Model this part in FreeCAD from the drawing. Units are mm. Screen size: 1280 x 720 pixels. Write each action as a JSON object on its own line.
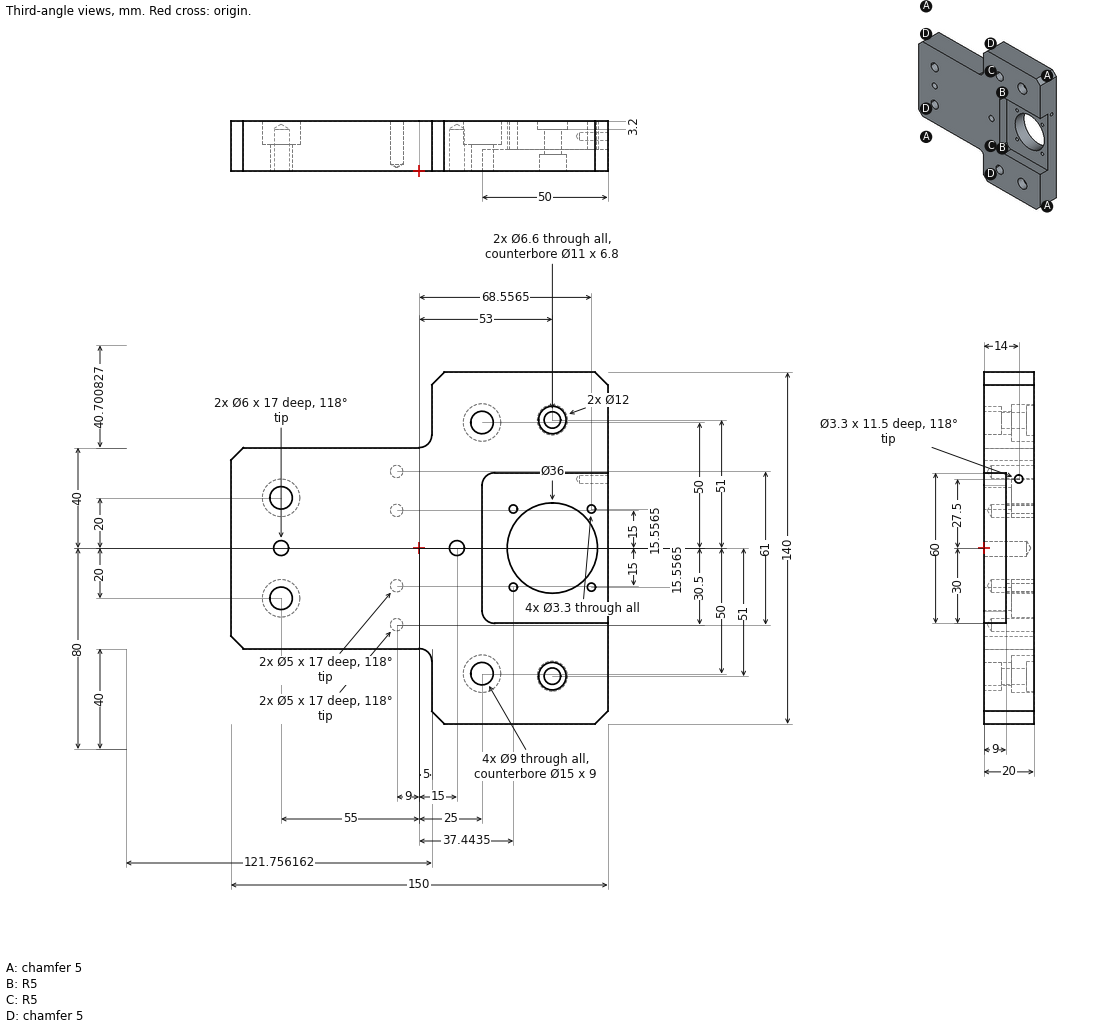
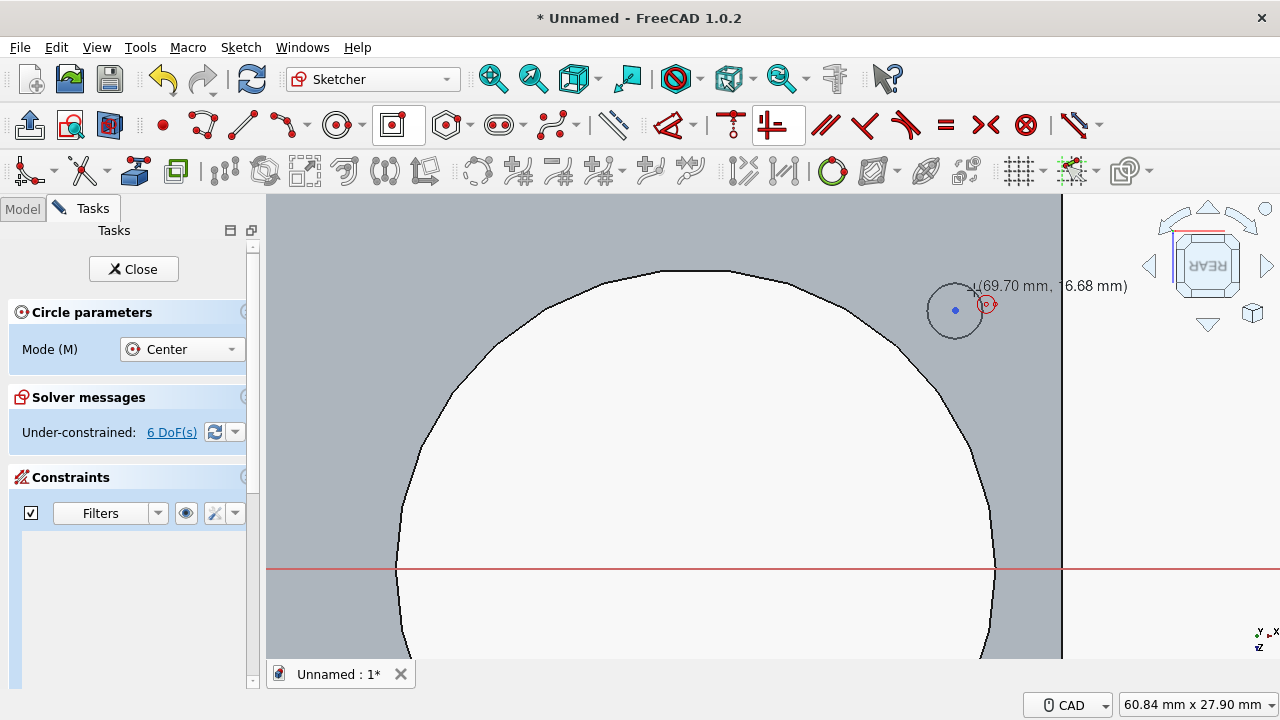
{"action": "left_click", "coordinate": [436, 310]}
{"action": "left_click", "coordinate": [456, 290]}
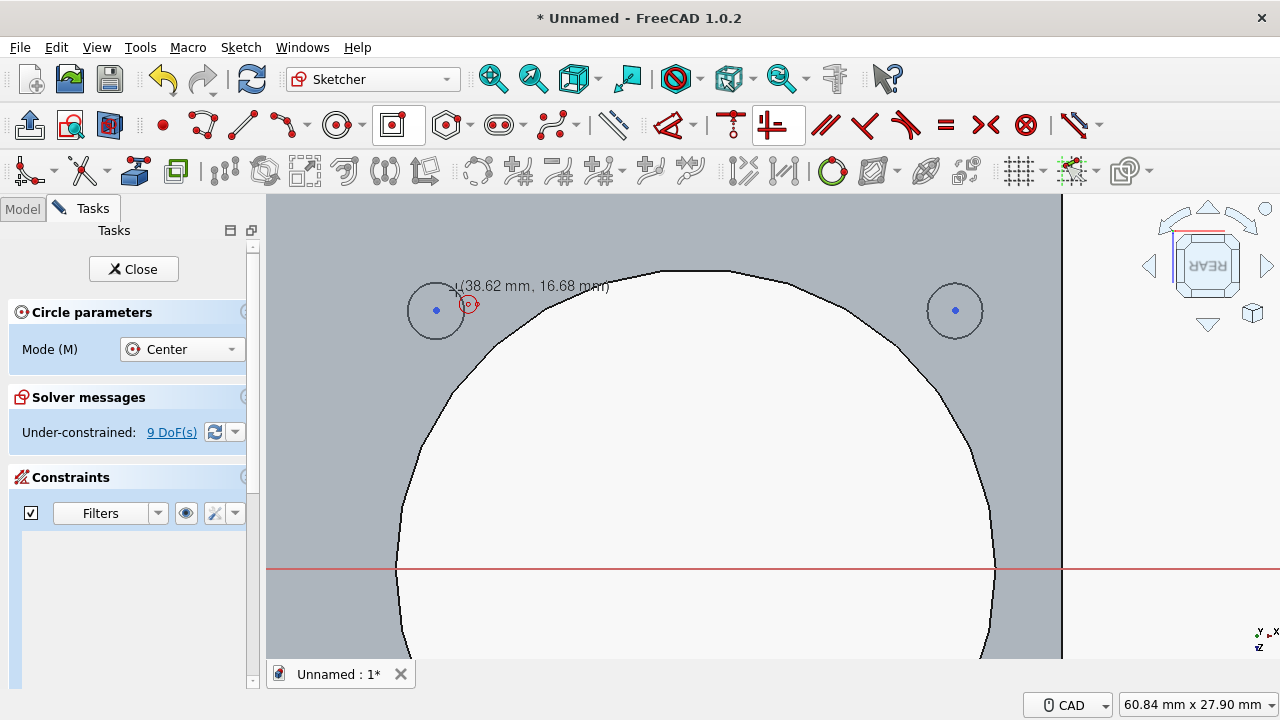
{"action": "scroll", "coordinate": [955, 310], "scroll_direction": "down", "scroll_amount": 4}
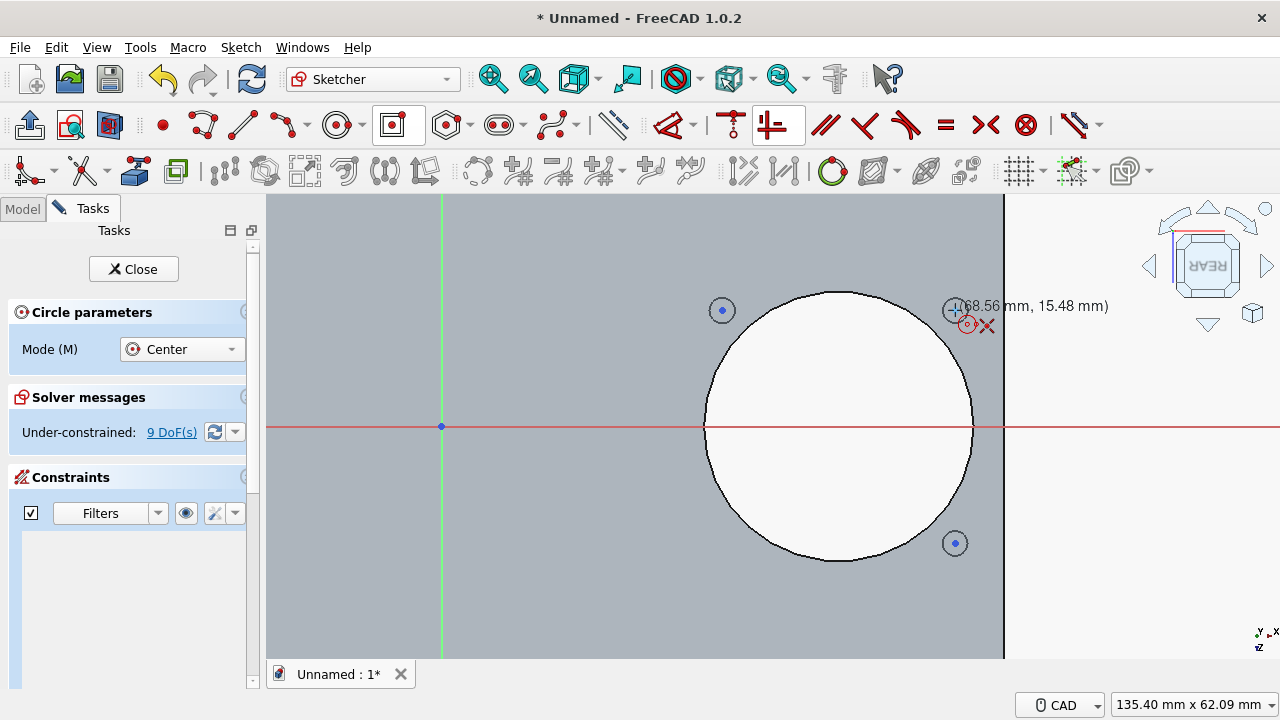
{"action": "scroll", "coordinate": [722, 543], "scroll_direction": "up", "scroll_amount": 4}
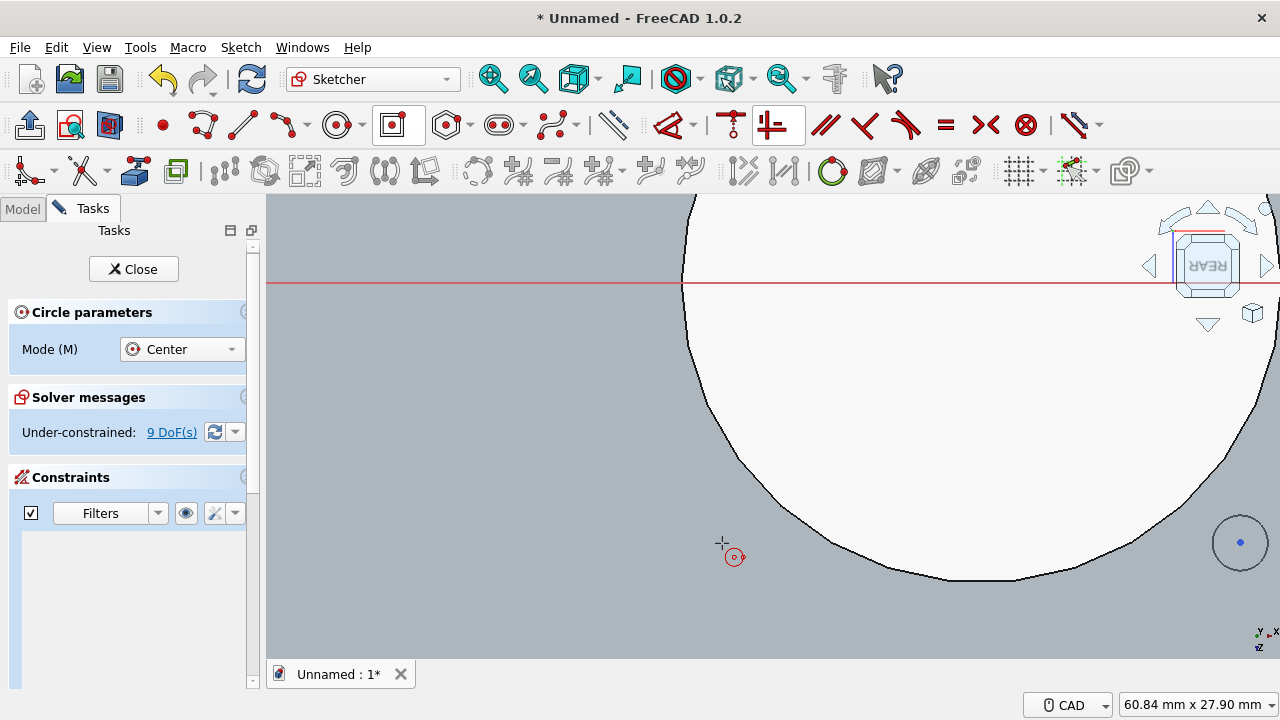
{"action": "left_click", "coordinate": [722, 542]}
{"action": "left_click", "coordinate": [742, 523]}
{"action": "key", "text": "Escape"}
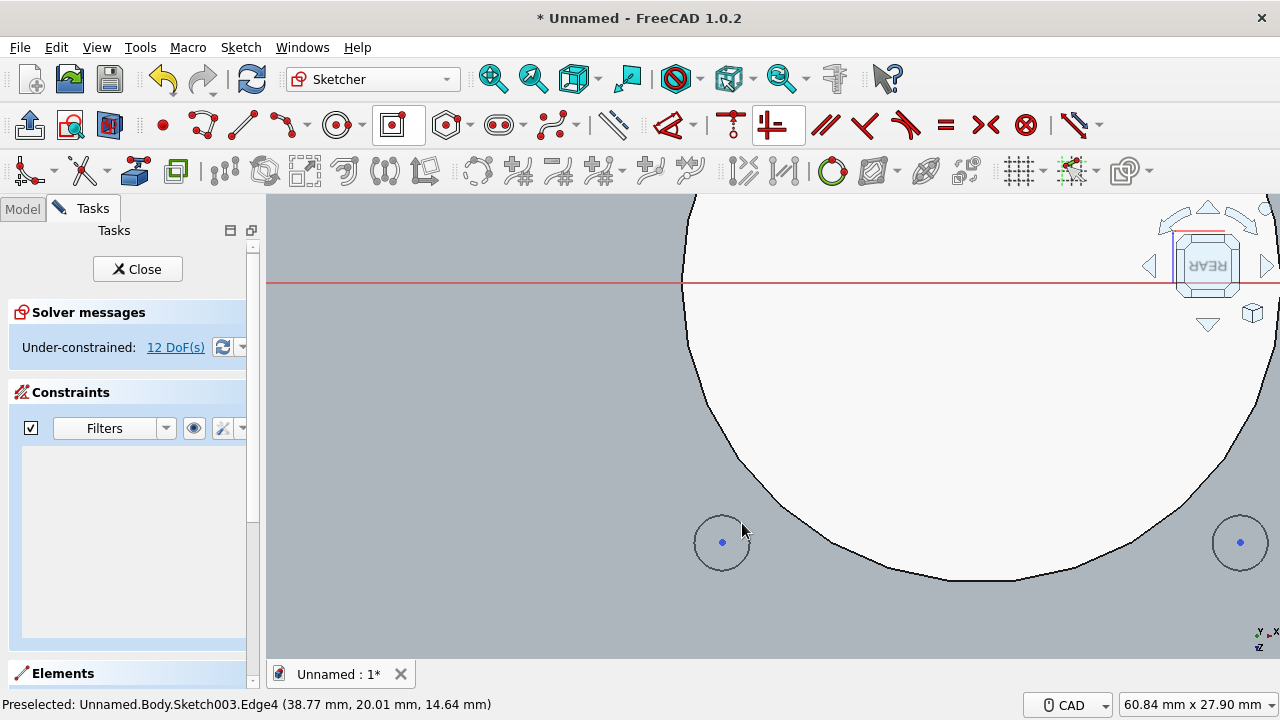
{"action": "scroll", "coordinate": [722, 544], "scroll_direction": "down", "scroll_amount": 4}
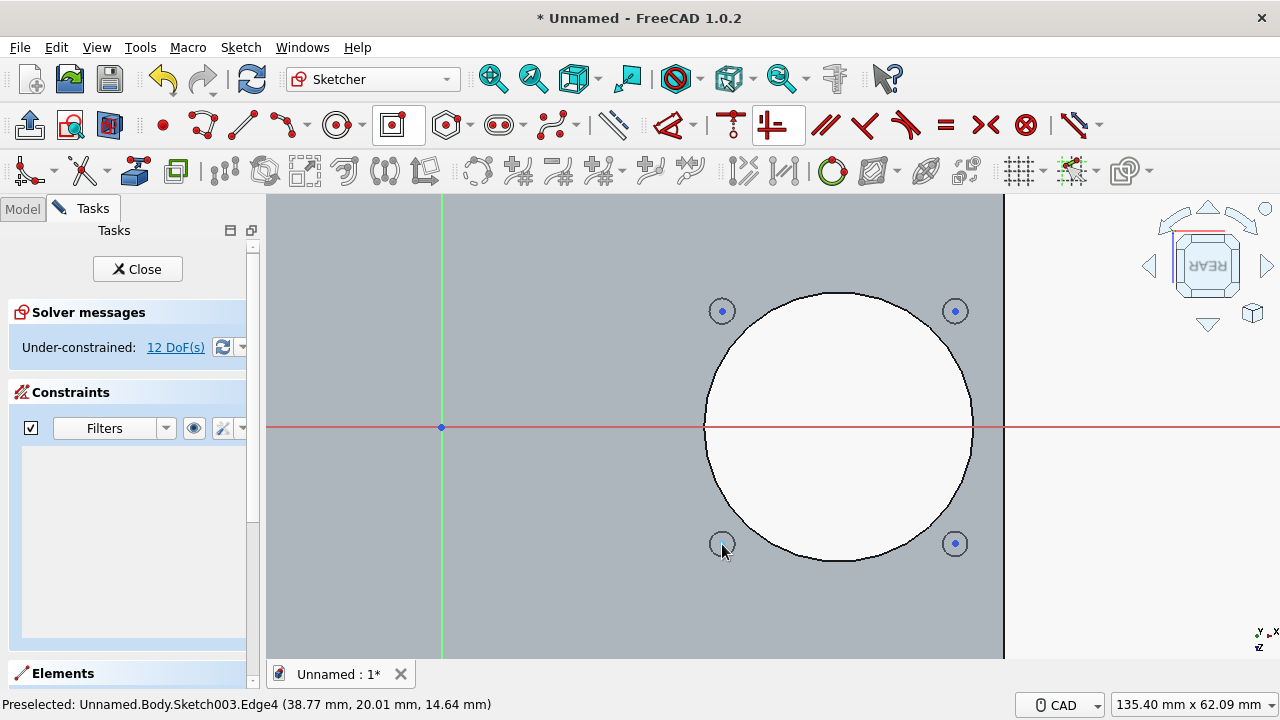
{"action": "left_click", "coordinate": [964, 535]}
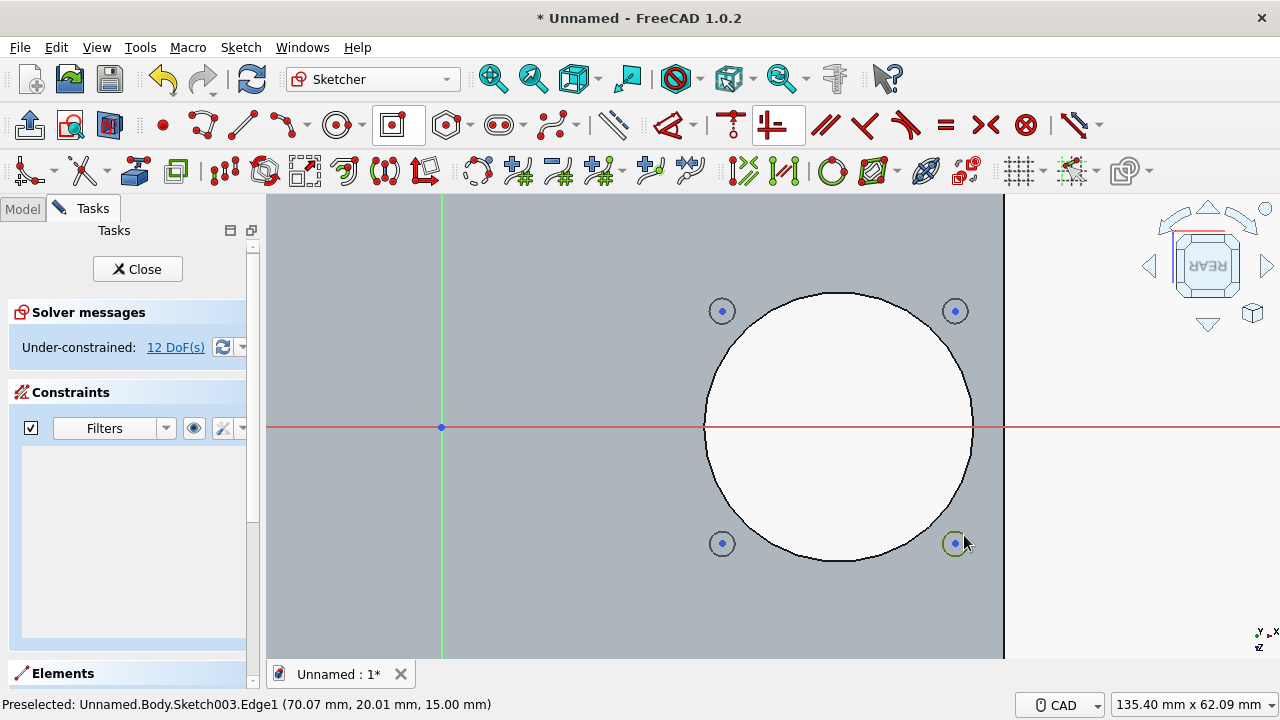
{"action": "left_click", "coordinate": [964, 302]}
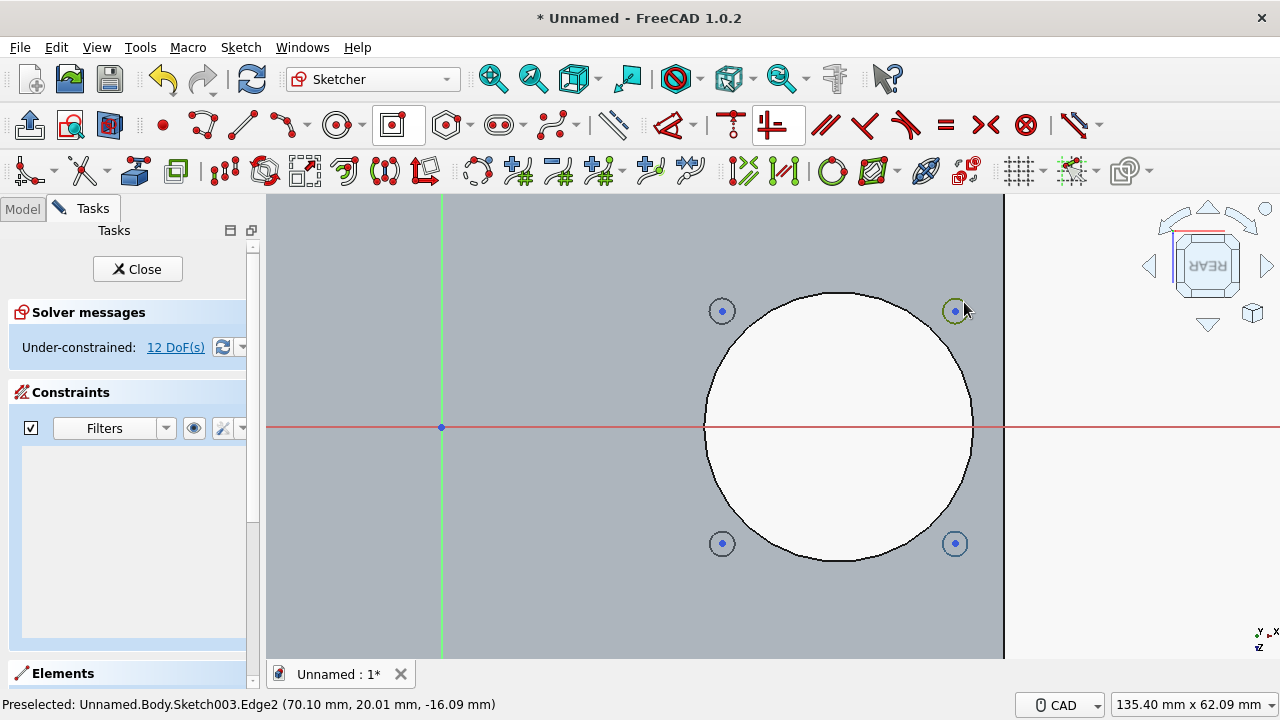
{"action": "left_click", "coordinate": [731, 302]}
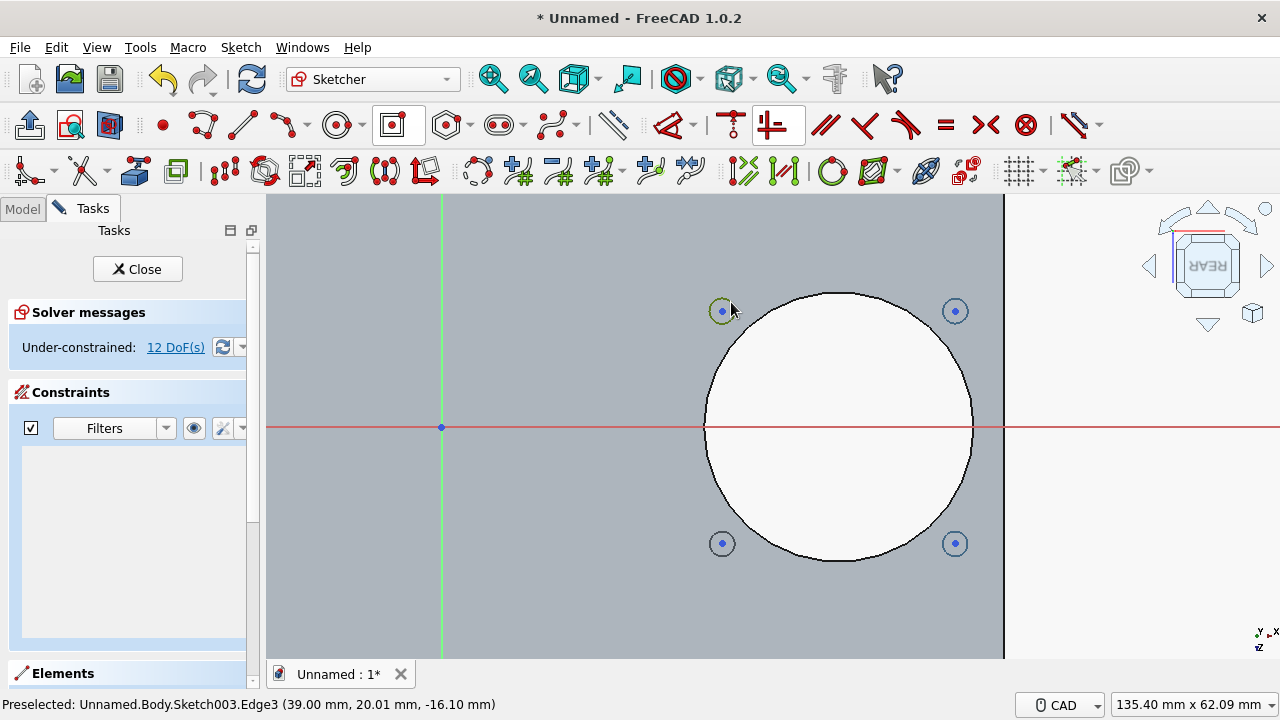
{"action": "left_click", "coordinate": [731, 535]}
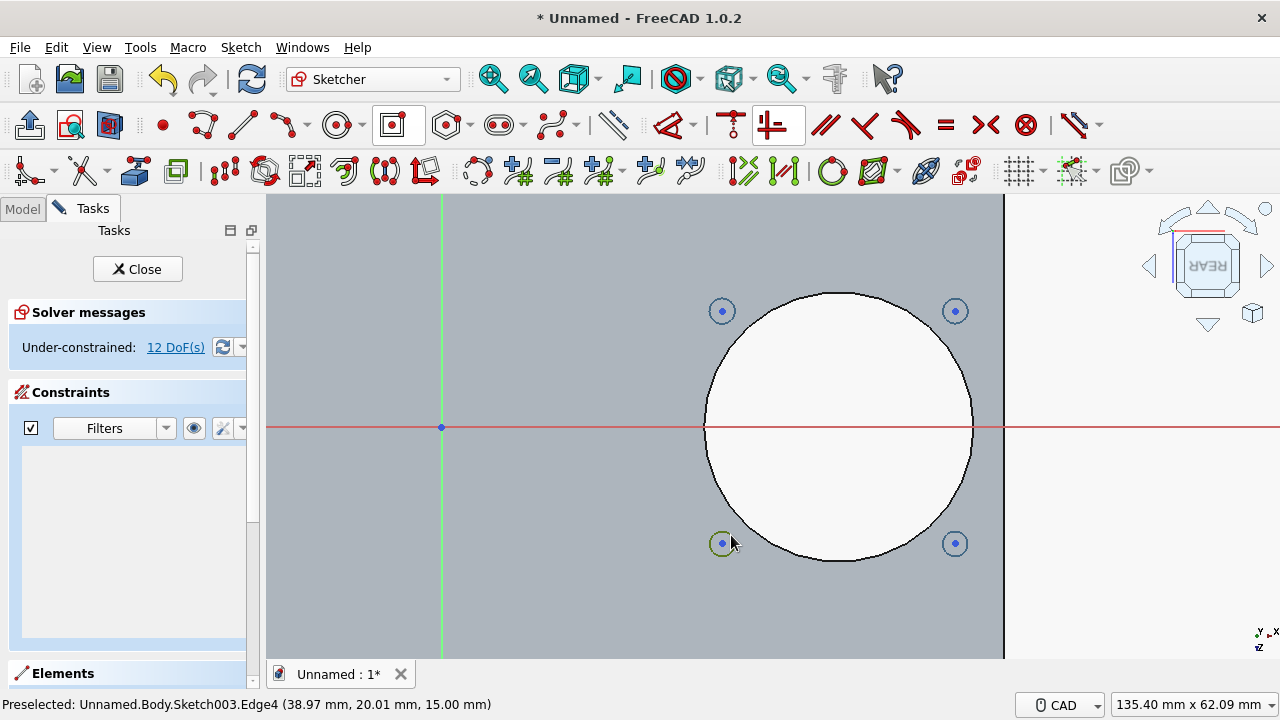
{"action": "left_click", "coordinate": [946, 126]}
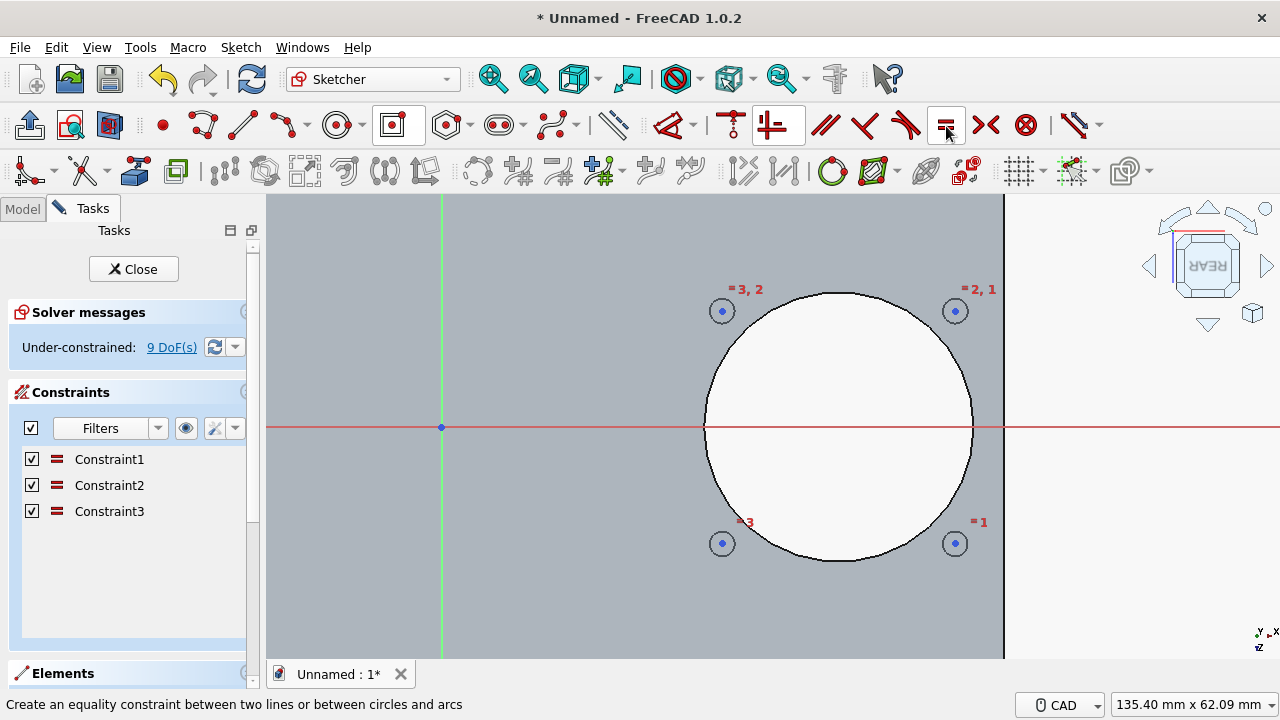
{"action": "left_click", "coordinate": [955, 544]}